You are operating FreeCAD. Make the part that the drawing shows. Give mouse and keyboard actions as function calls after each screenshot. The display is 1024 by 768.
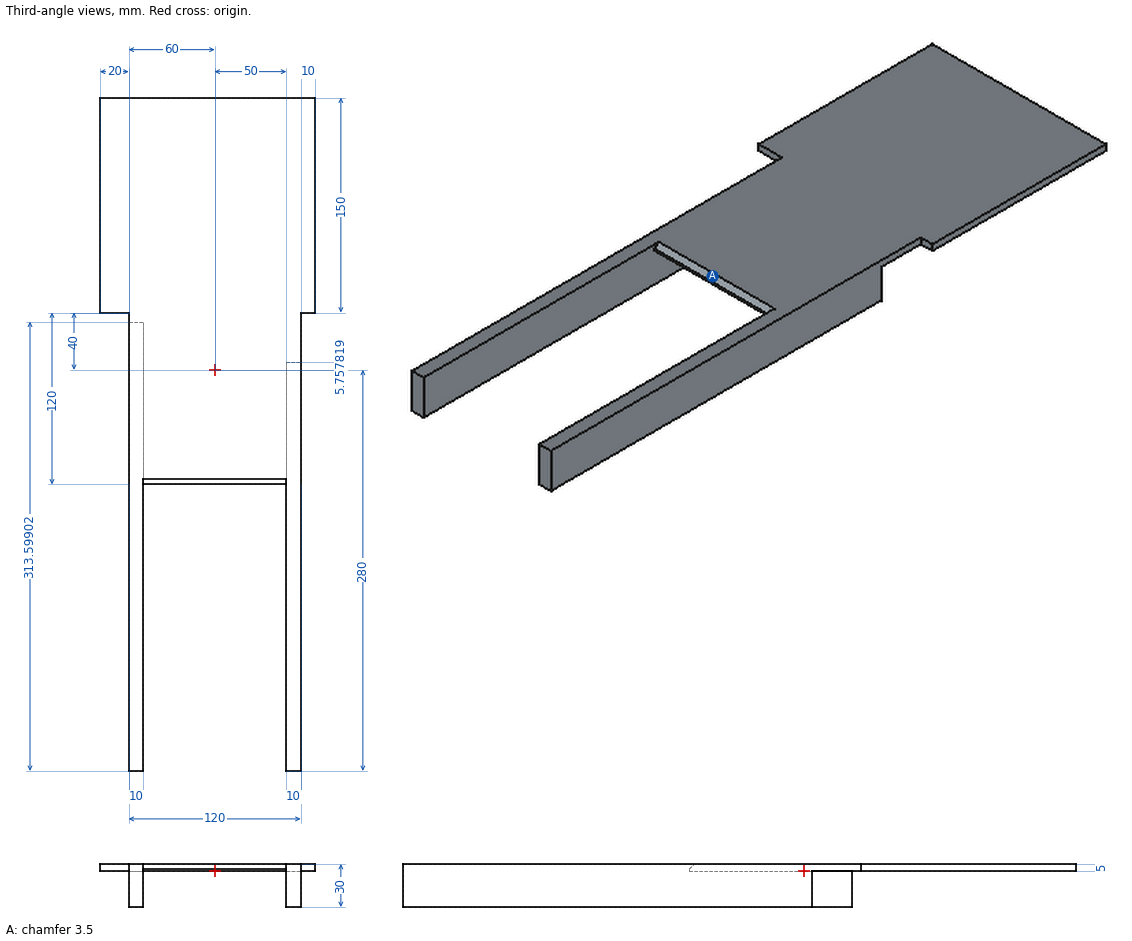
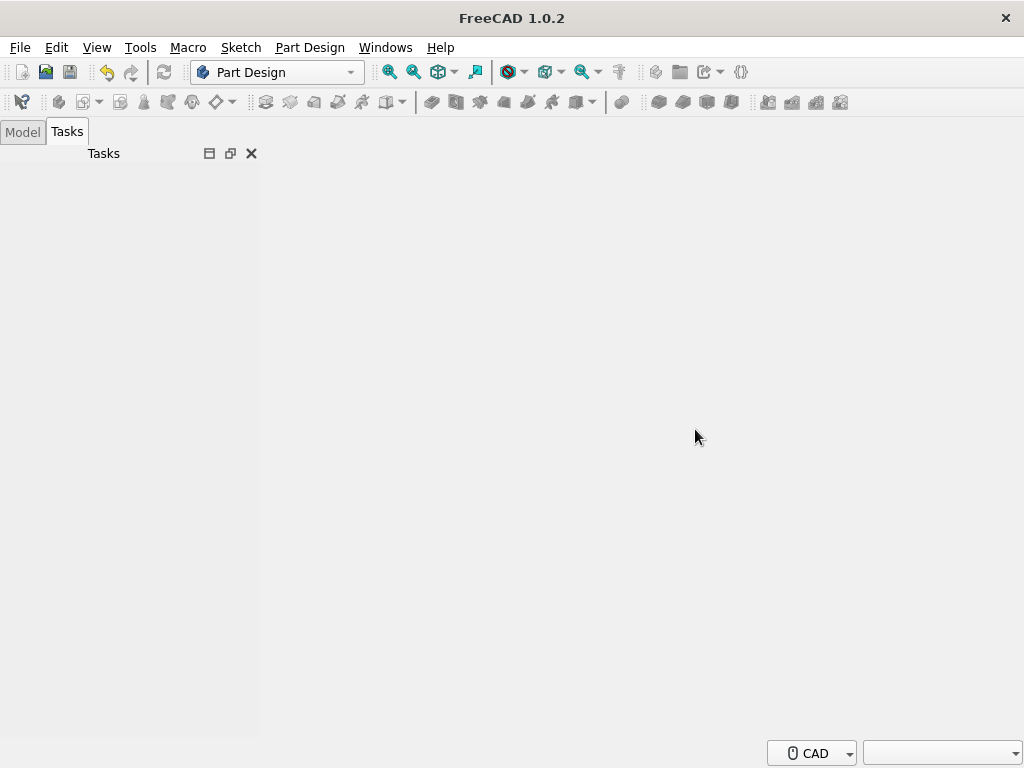
click(22, 72)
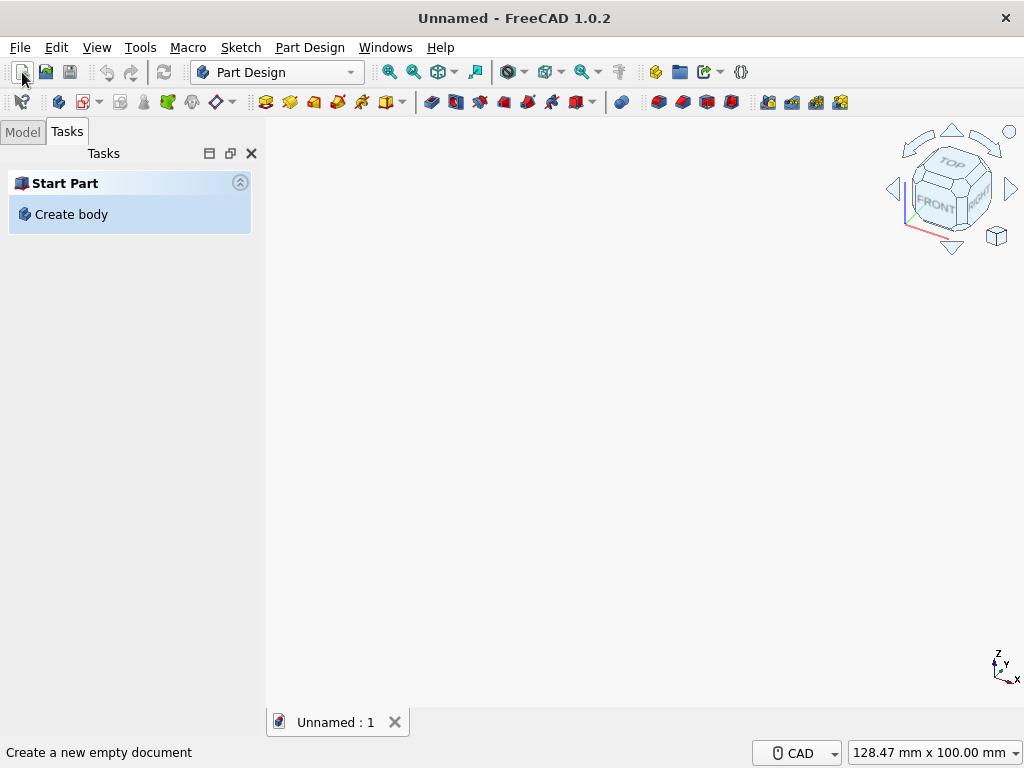
click(84, 102)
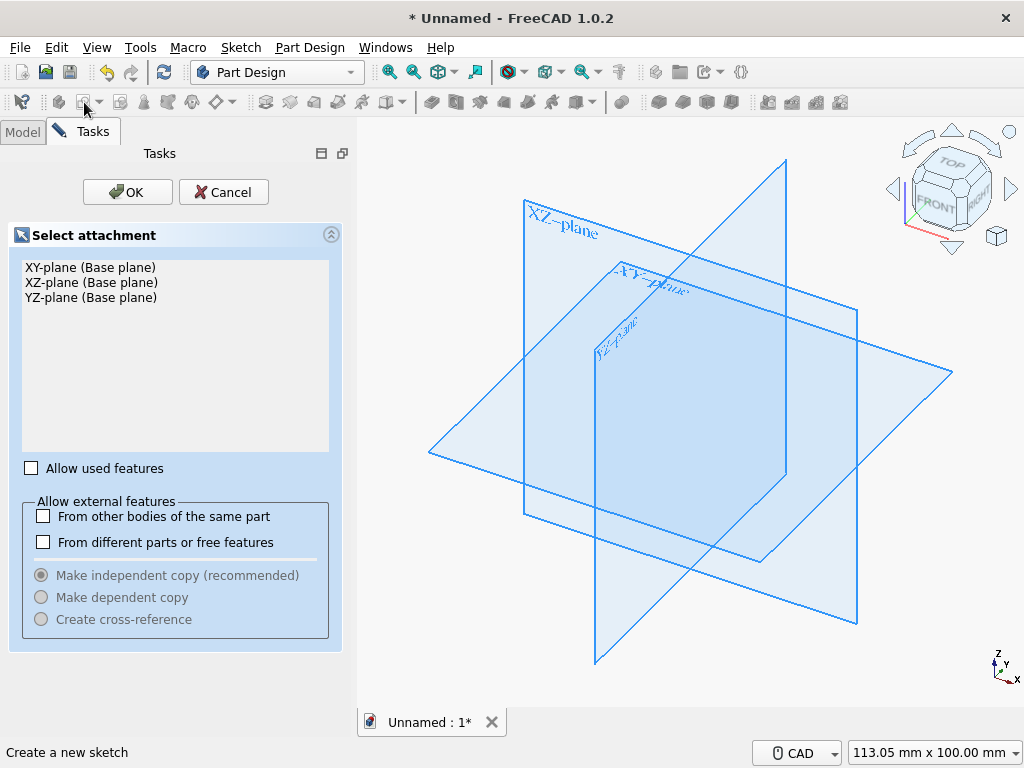
click(82, 268)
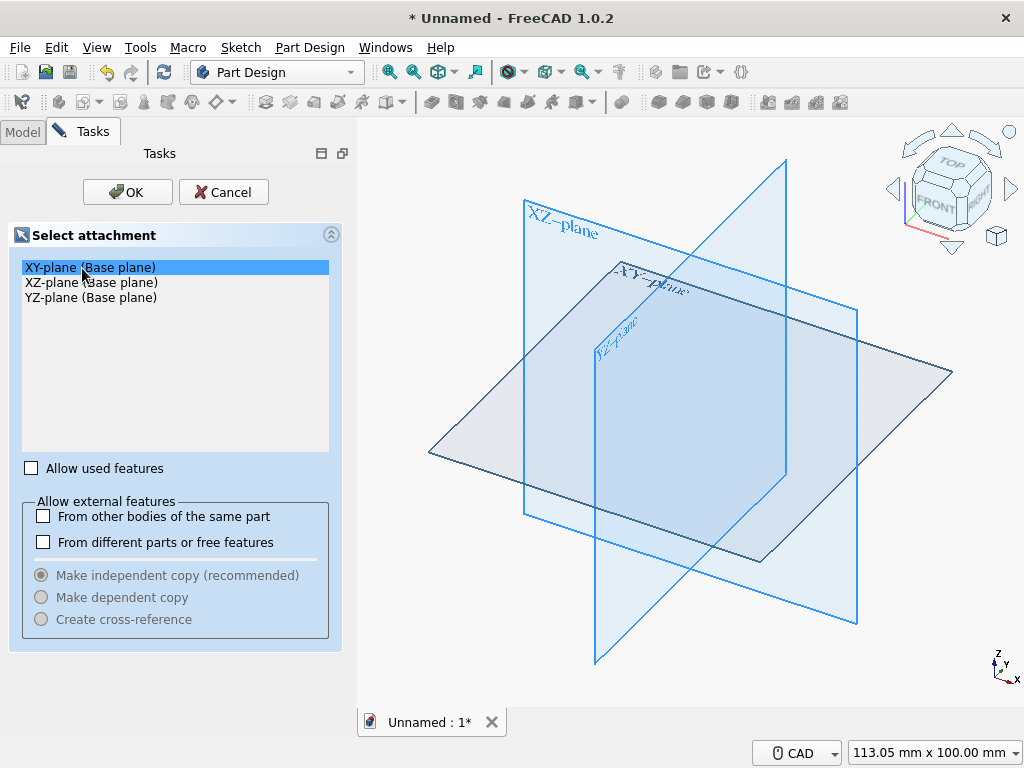
click(128, 192)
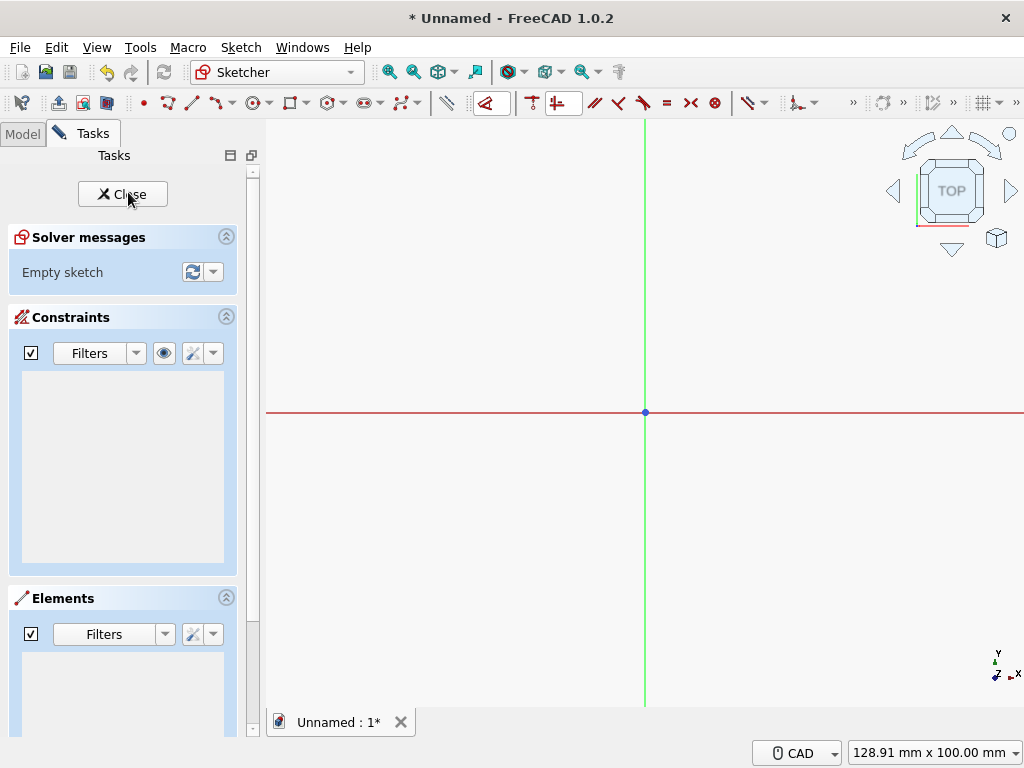
scroll(564, 519, down, 7)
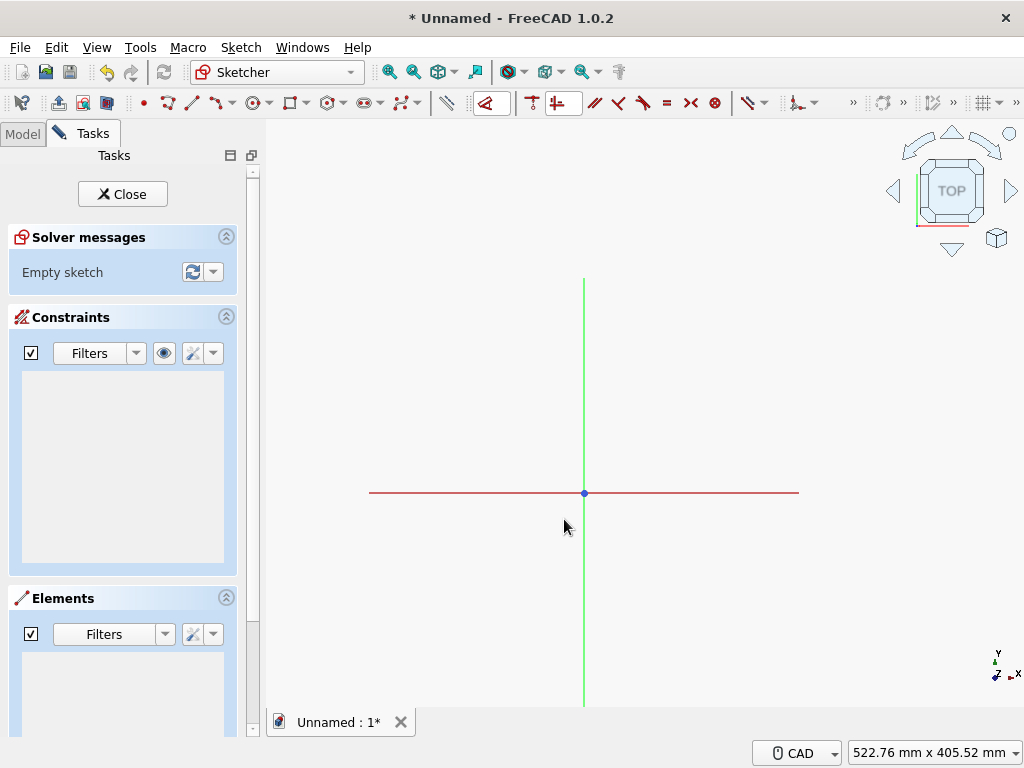
click(168, 104)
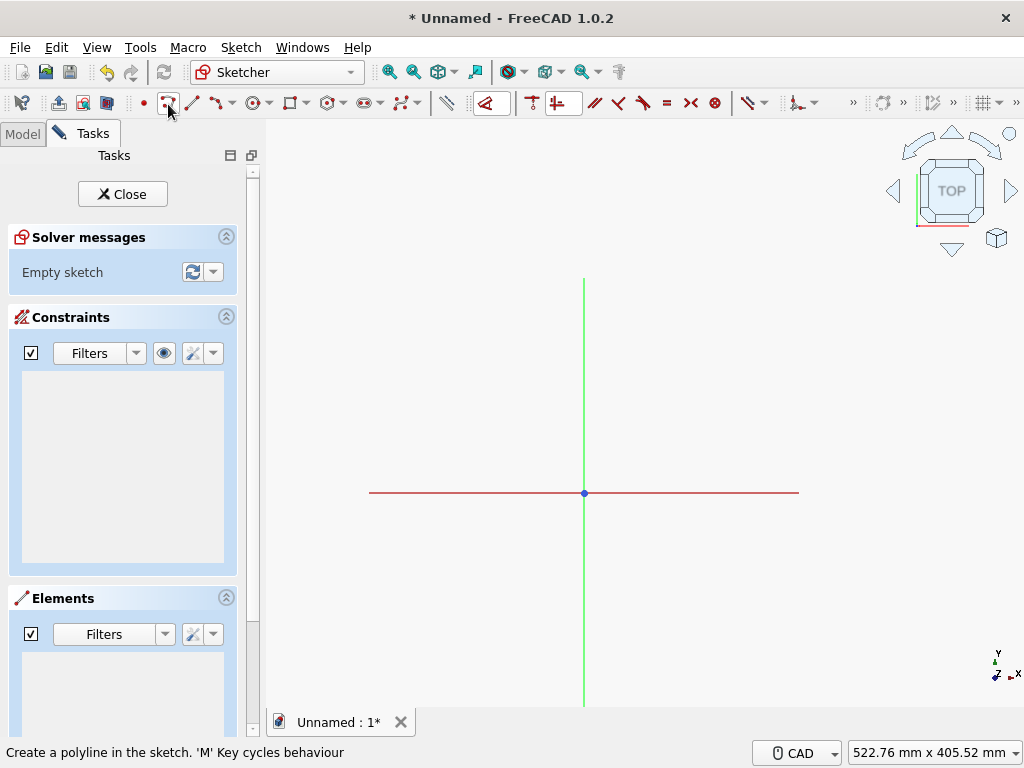
click(497, 435)
click(497, 609)
click(671, 609)
click(671, 435)
click(686, 435)
click(686, 218)
click(468, 218)
click(468, 435)
click(497, 436)
key(Escape)
key(Escape)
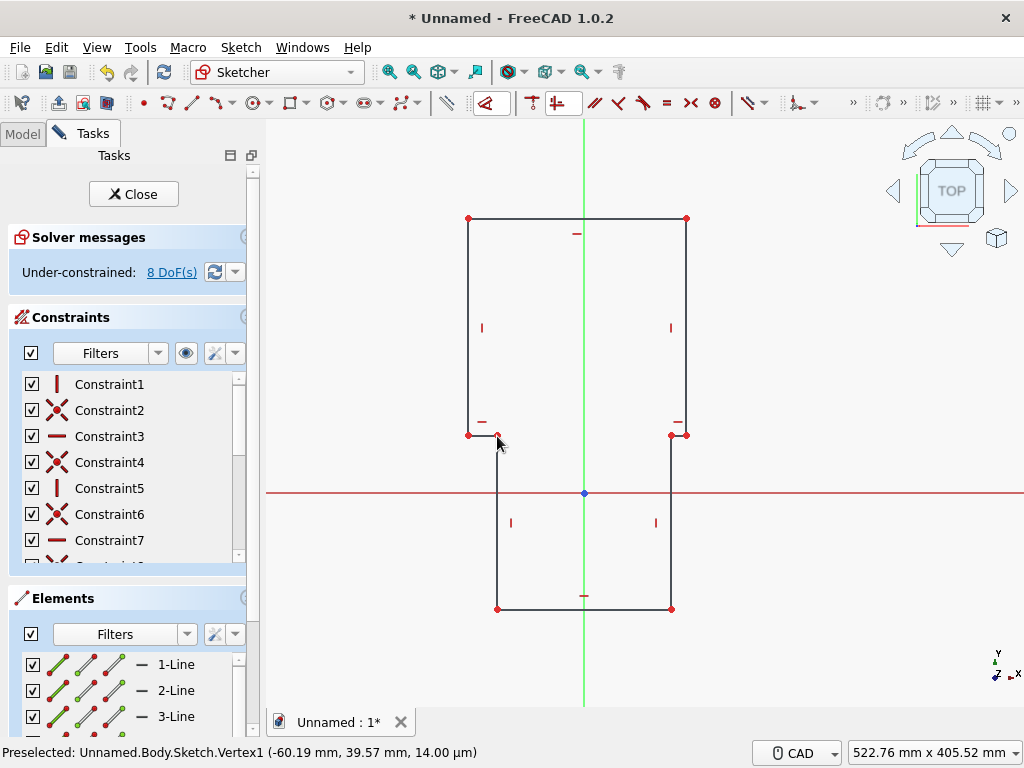
click(486, 104)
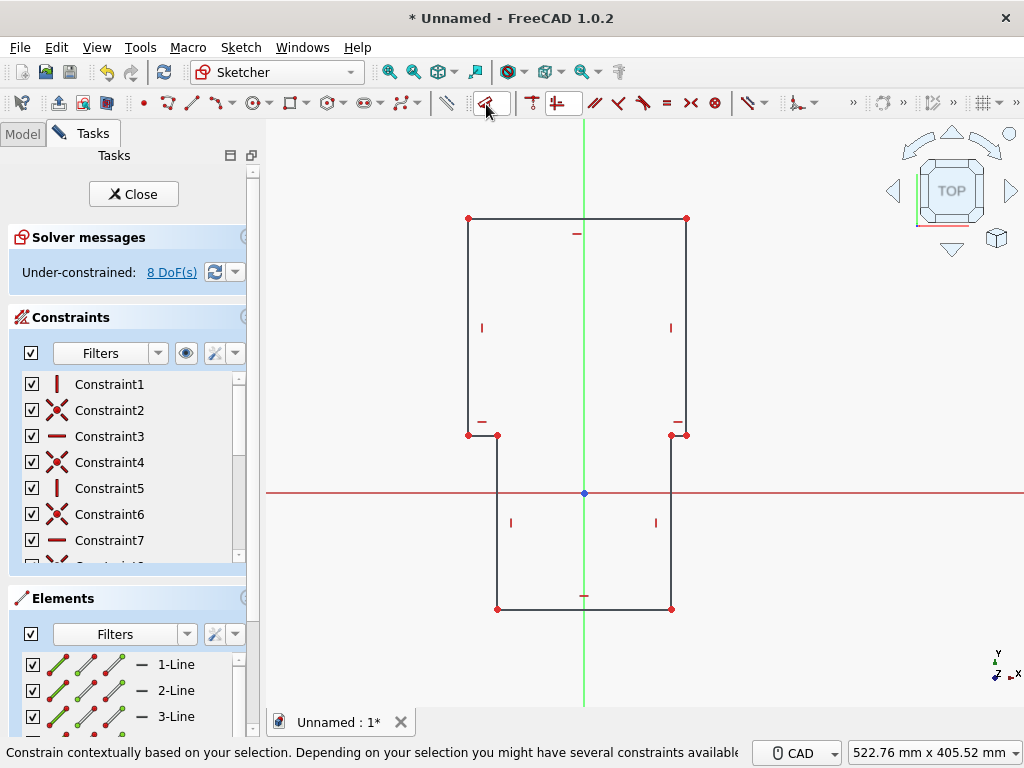
scroll(679, 436, up, 6)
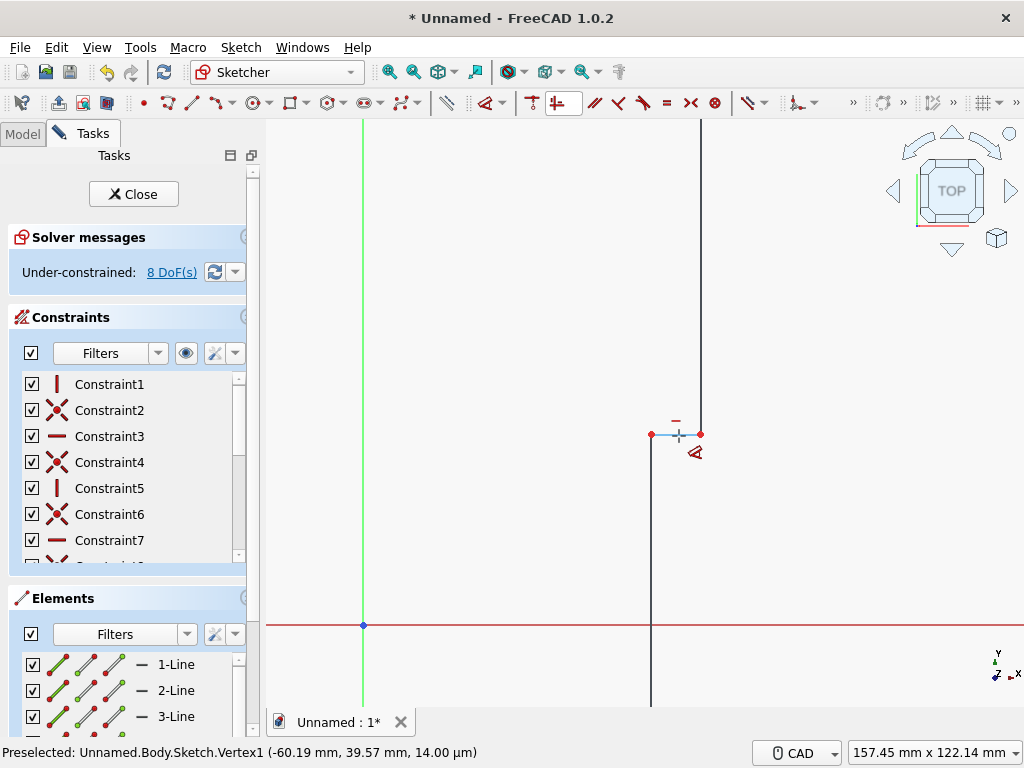
click(676, 435)
click(676, 469)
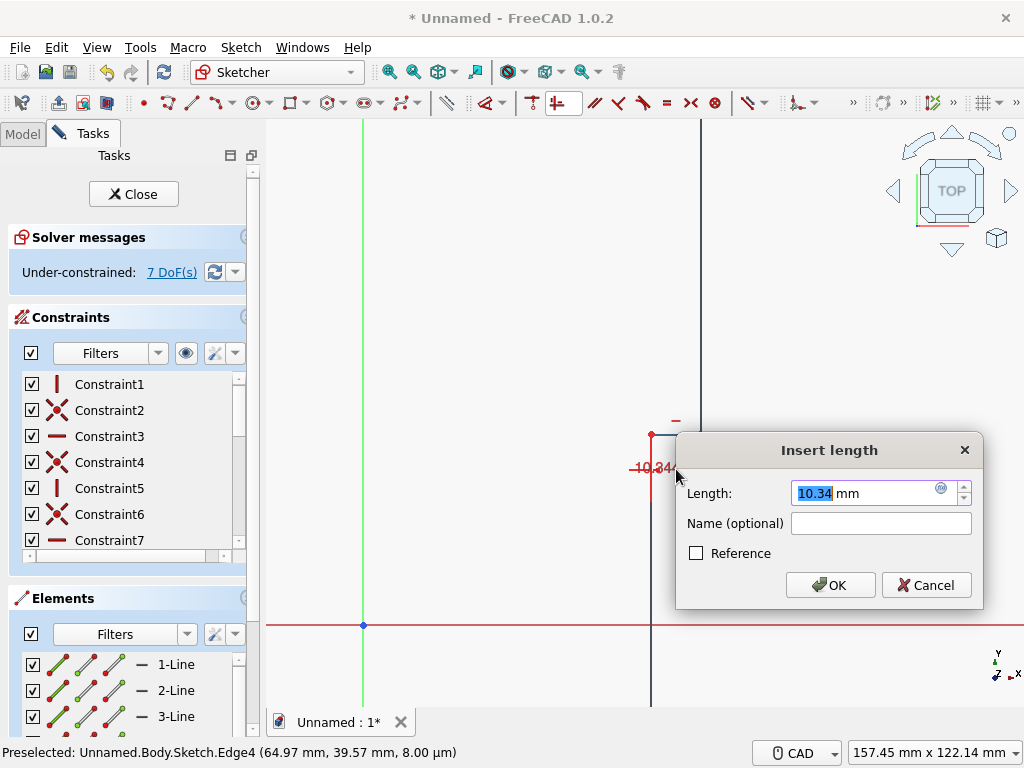
text(10)
key(Return)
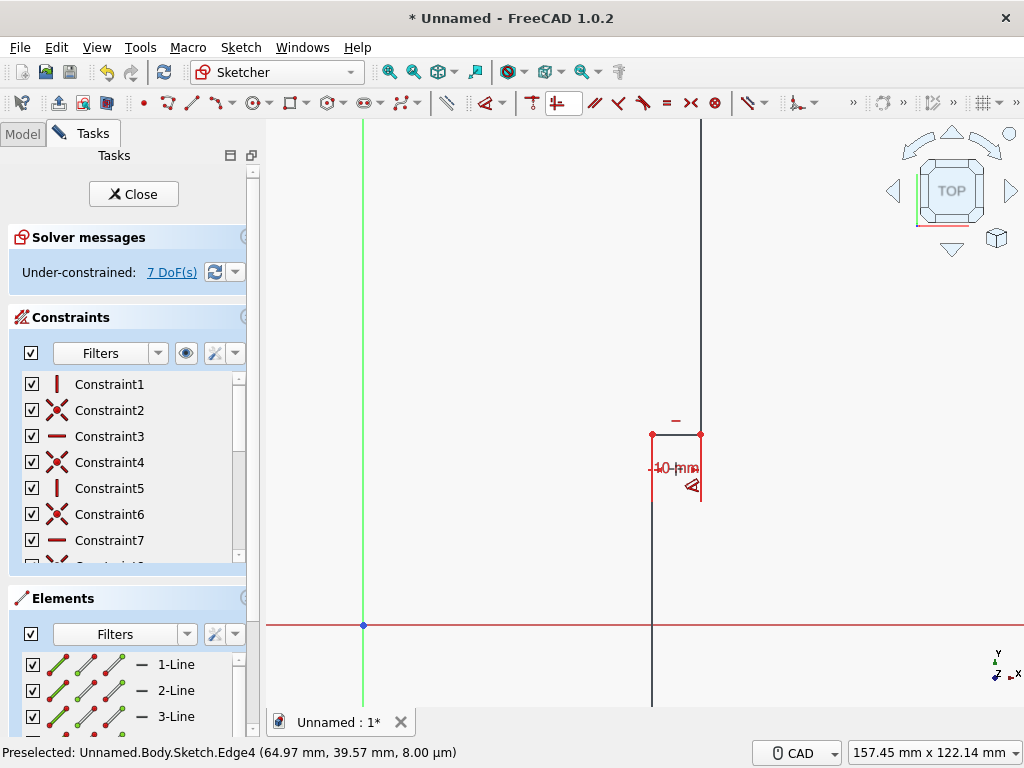
scroll(679, 436, down, 6)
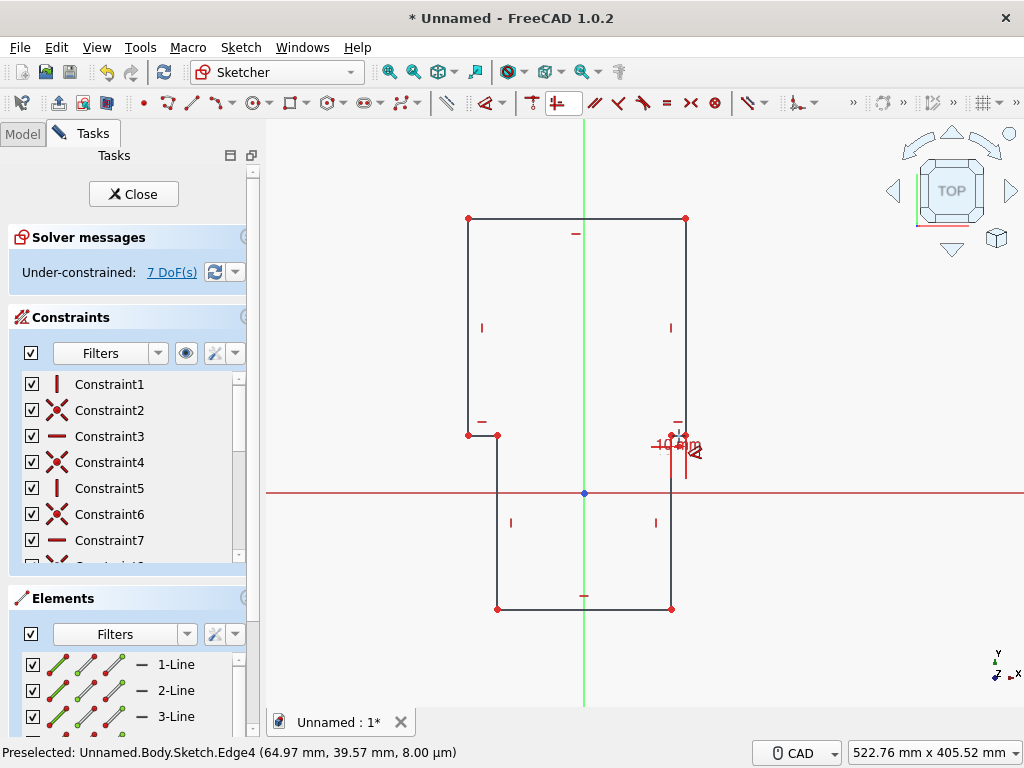
scroll(477, 436, up, 3)